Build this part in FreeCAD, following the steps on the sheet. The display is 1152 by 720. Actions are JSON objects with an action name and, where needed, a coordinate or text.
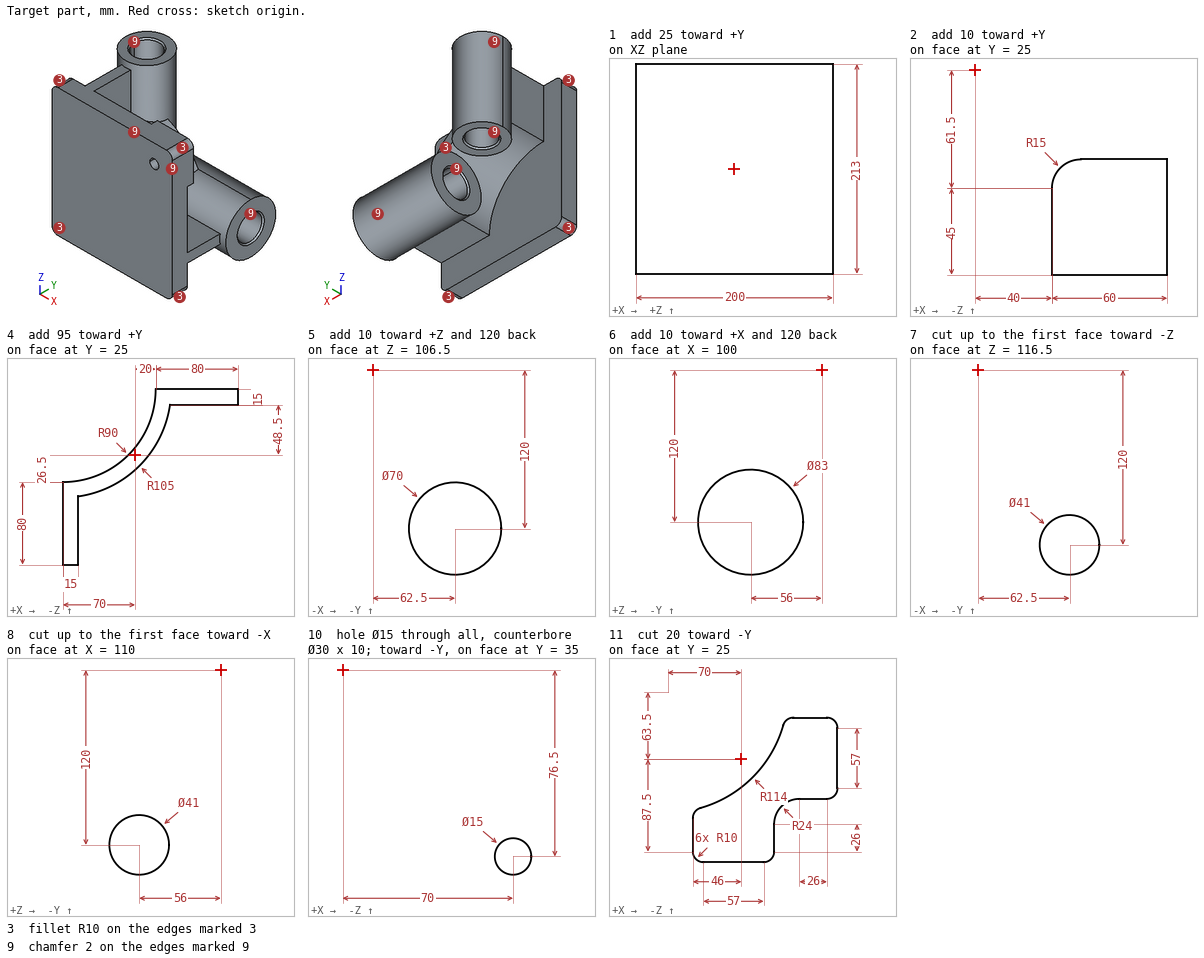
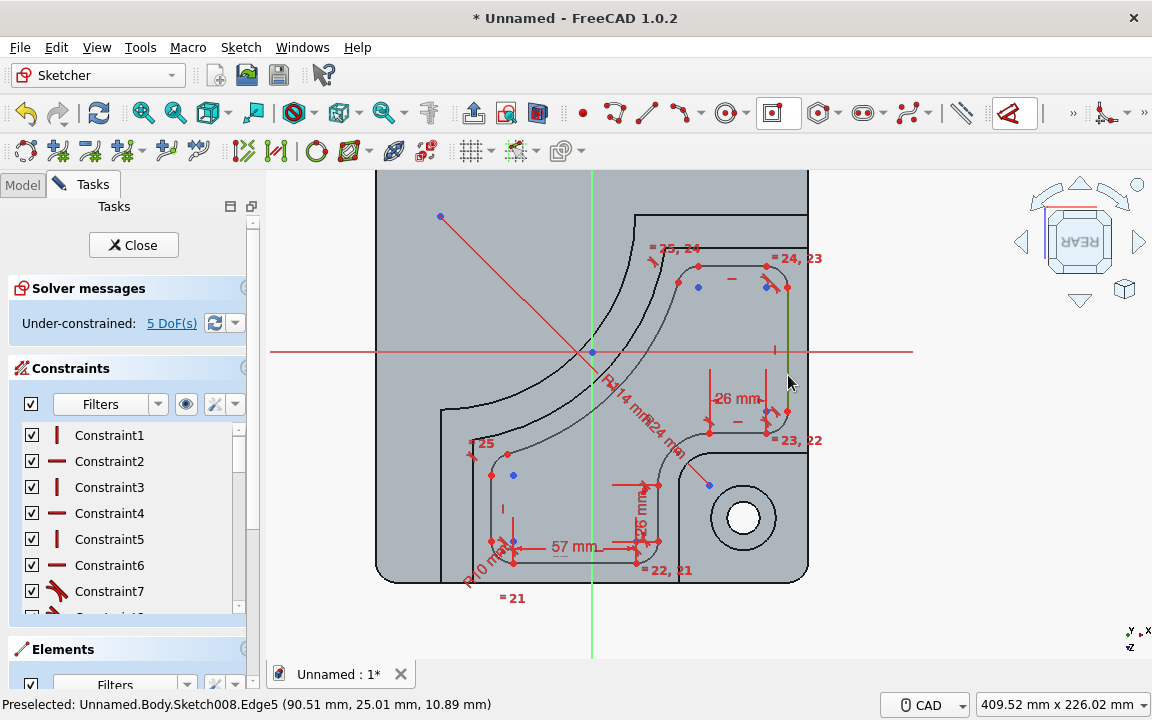
{"action": "left_click", "coordinate": [1032, 114]}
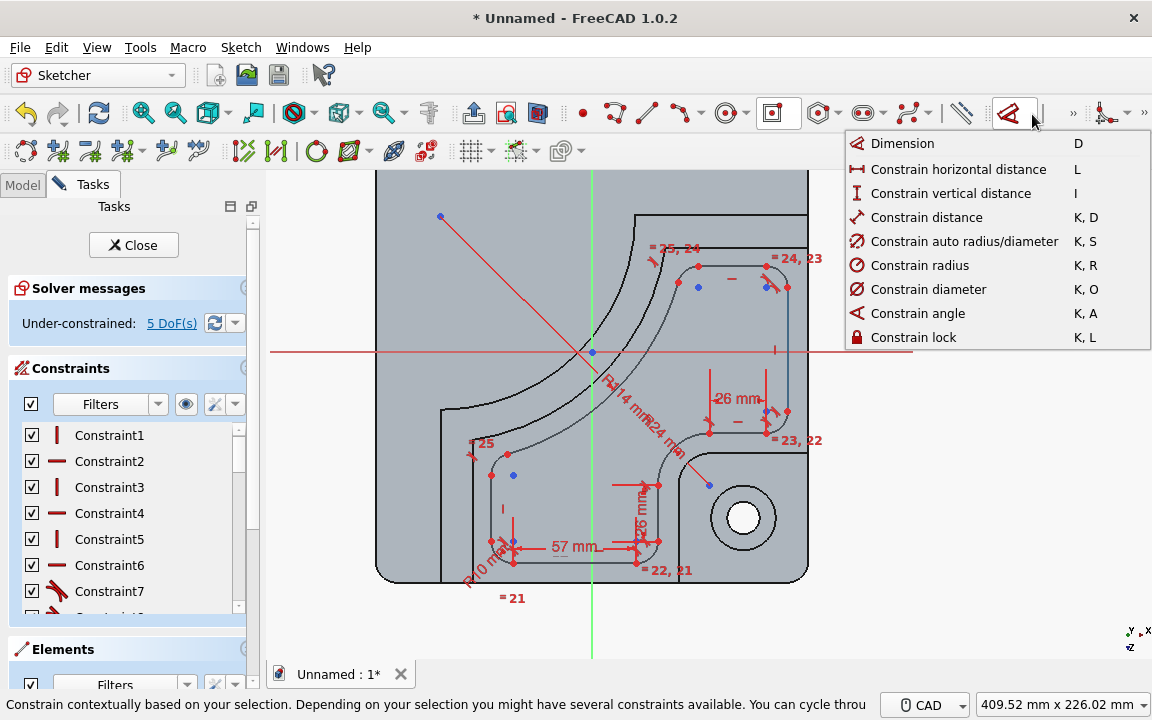
{"action": "left_click", "coordinate": [998, 193]}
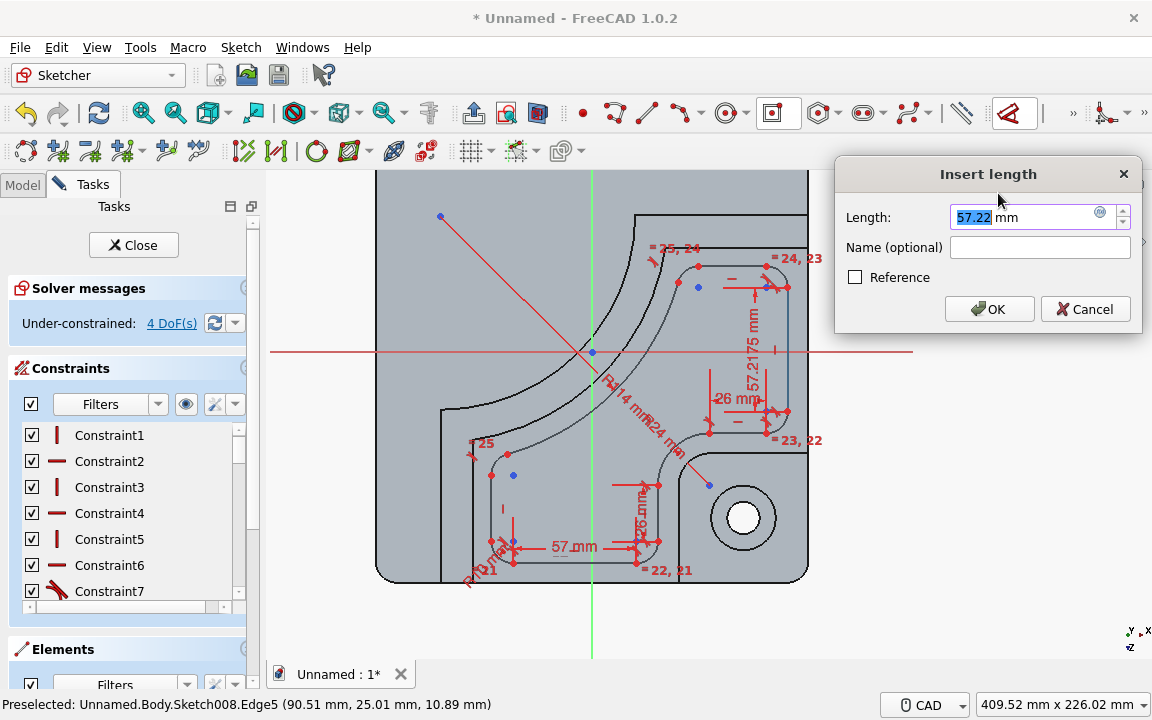
{"action": "type", "text": "57"}
{"action": "key", "text": "Return"}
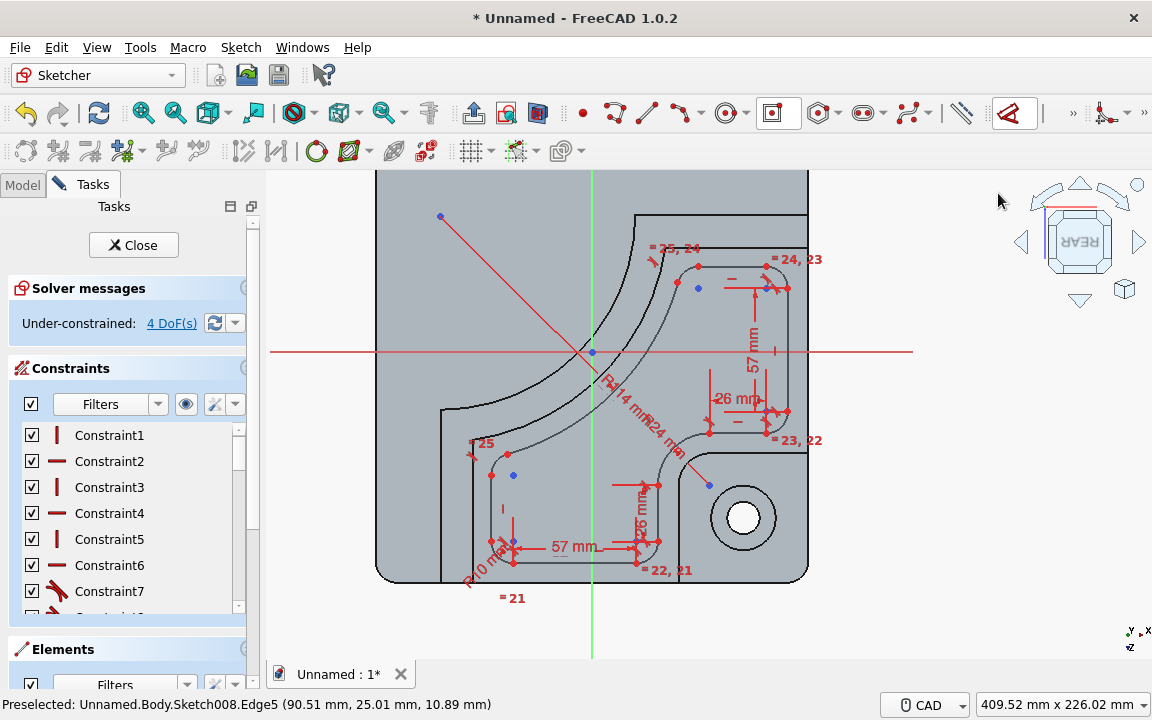
{"action": "left_click", "coordinate": [491, 475]}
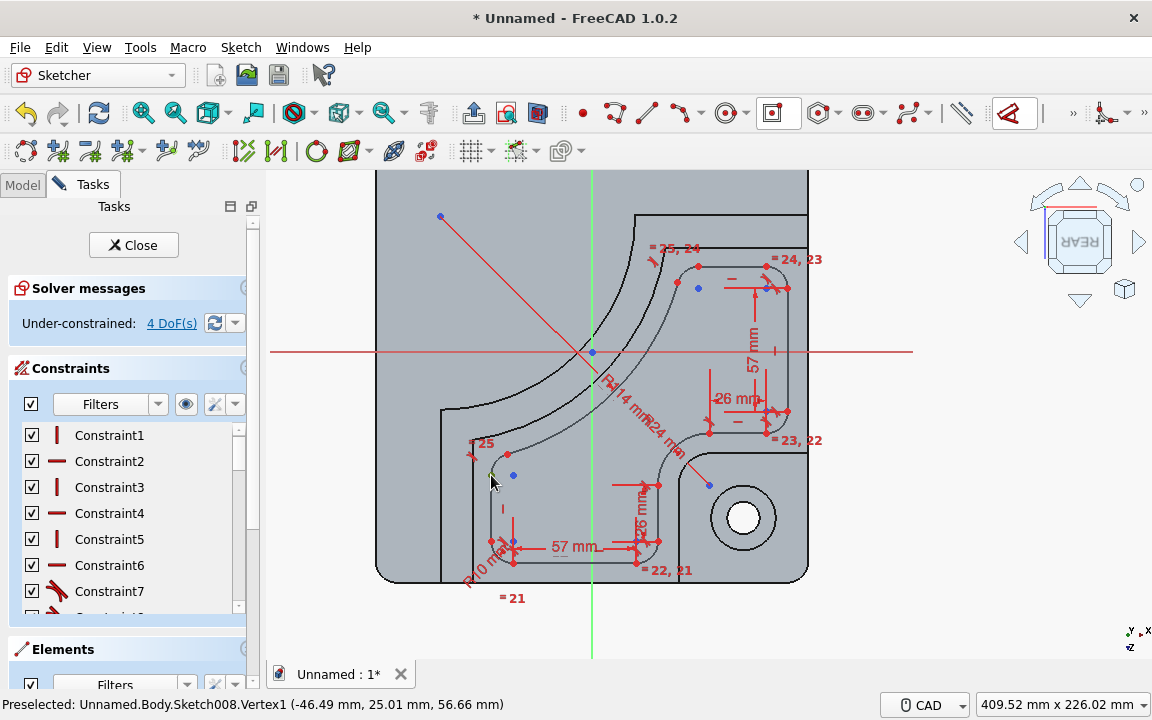
{"action": "key", "text": "l"}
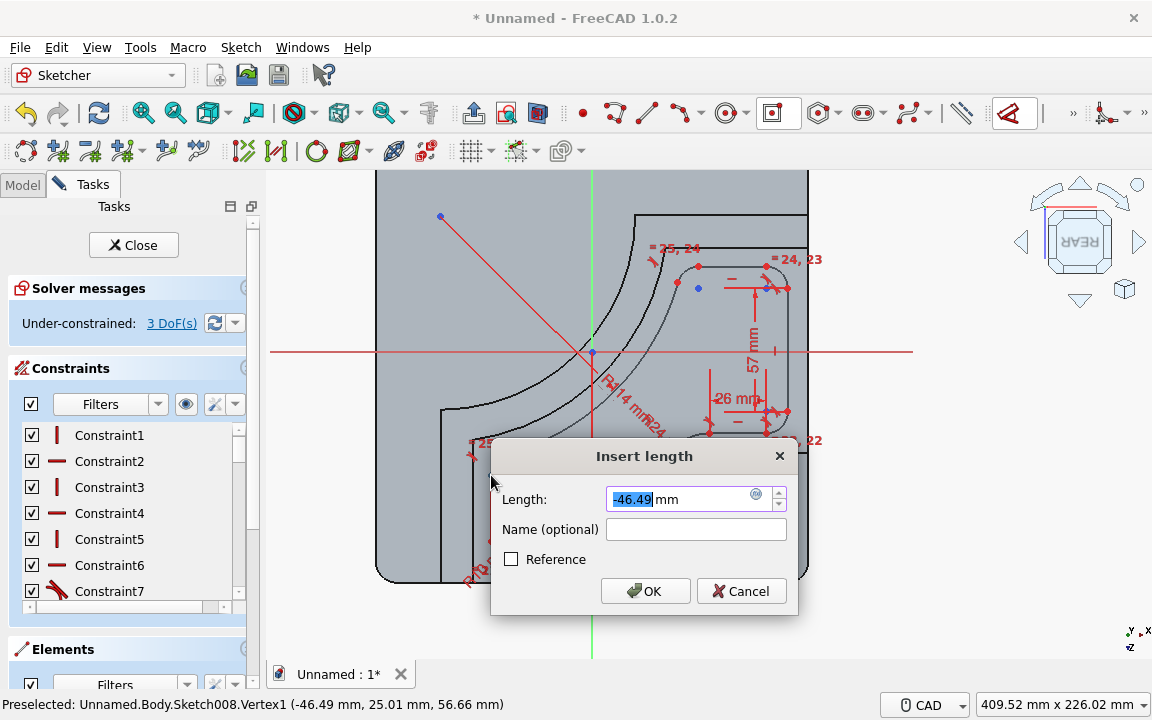
{"action": "type", "text": "-46"}
{"action": "key", "text": "Return"}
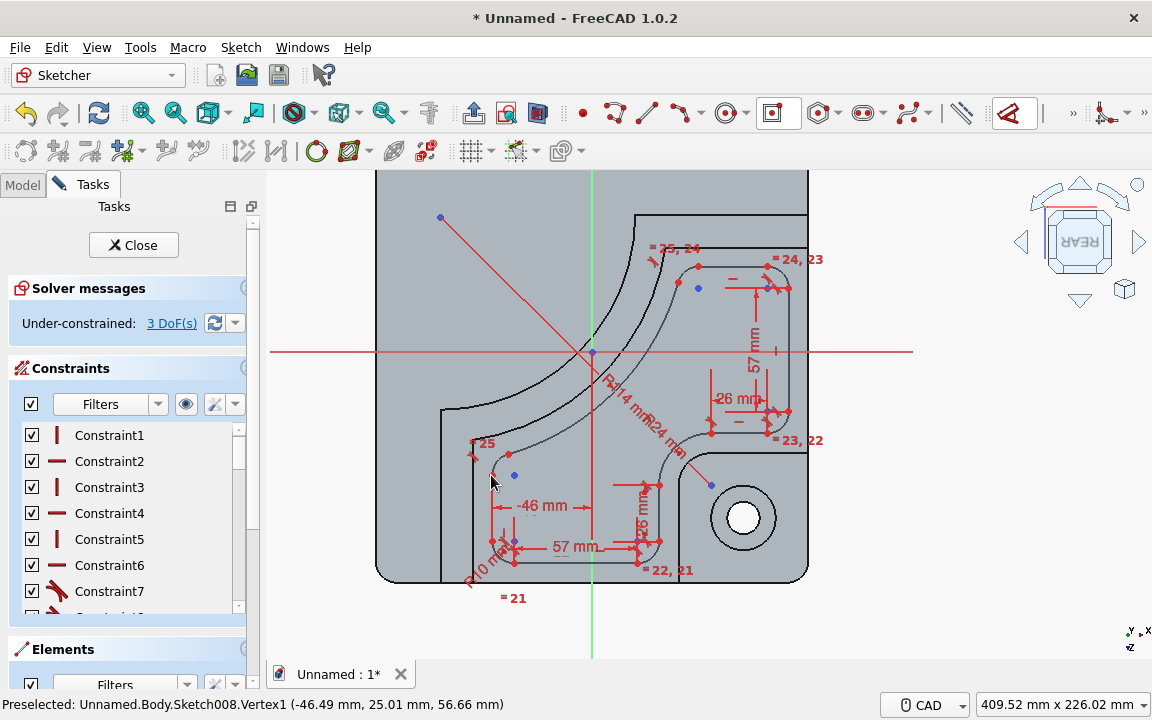
{"action": "left_click", "coordinate": [440, 217]}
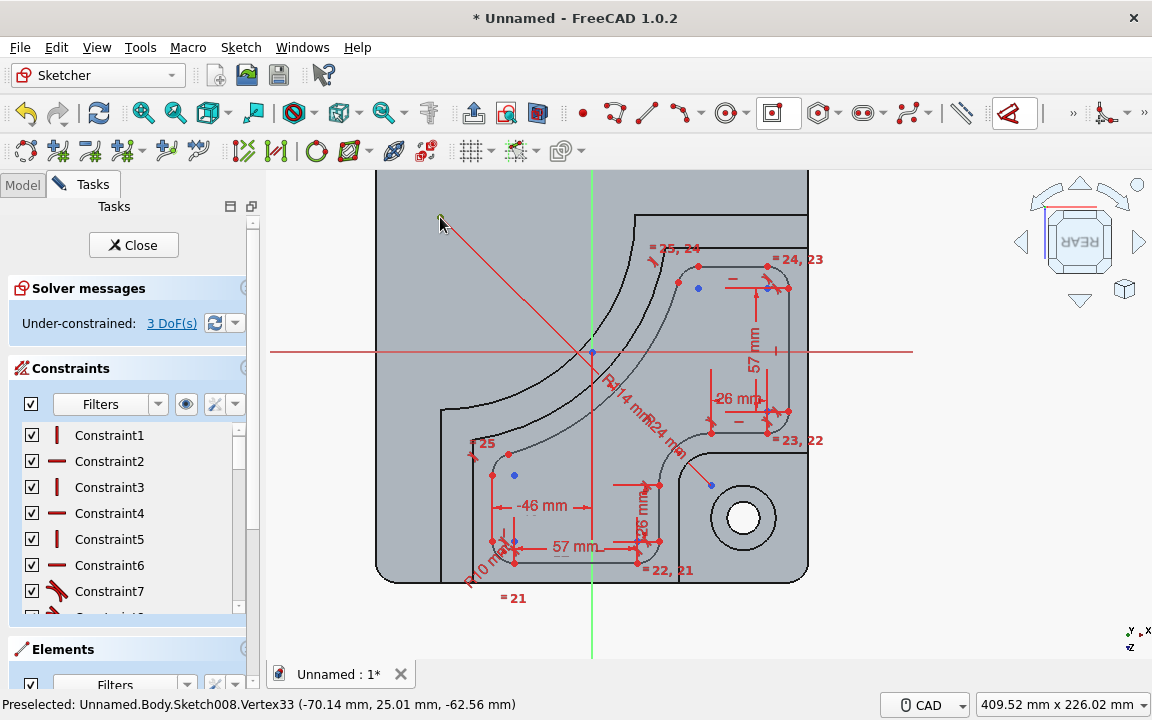
{"action": "key", "text": "l"}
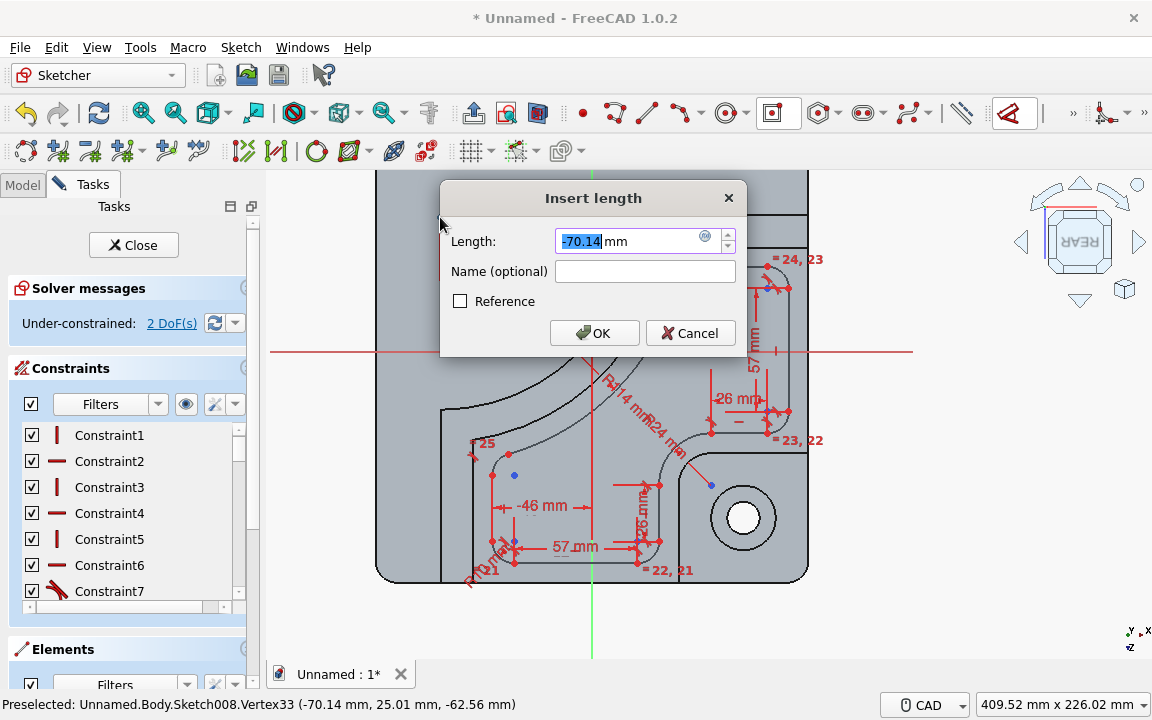
{"action": "type", "text": "-70"}
{"action": "key", "text": "Return"}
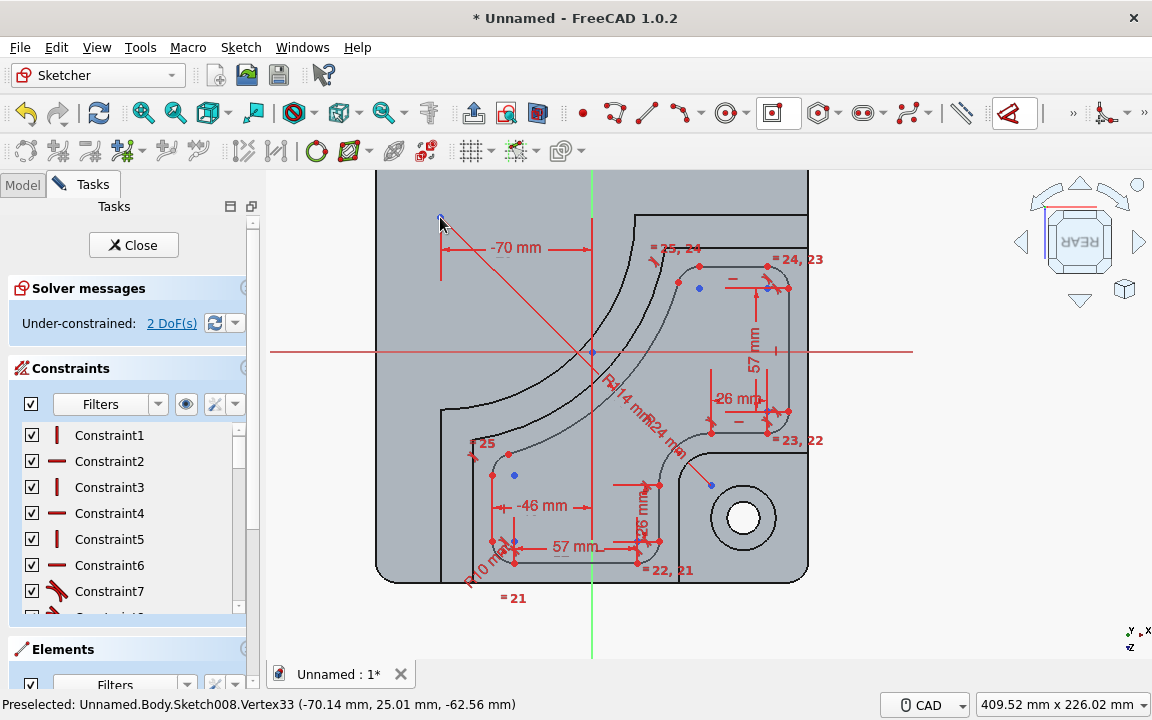
{"action": "left_click", "coordinate": [493, 542]}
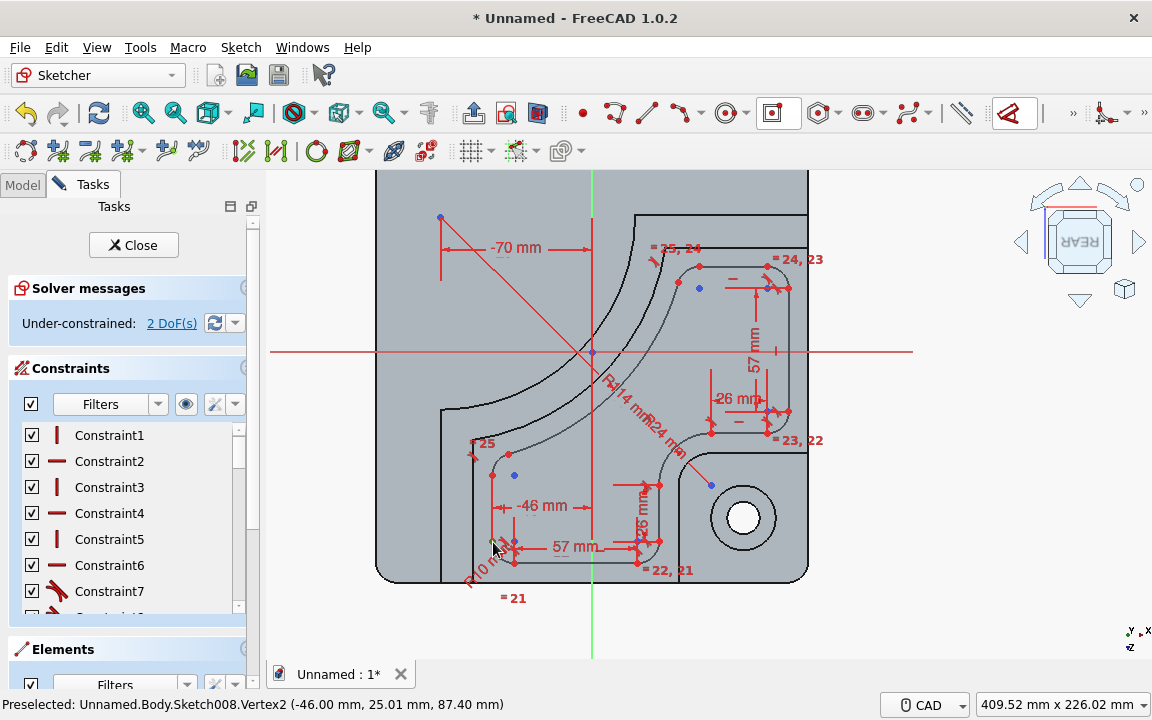
{"action": "left_click", "coordinate": [1032, 114]}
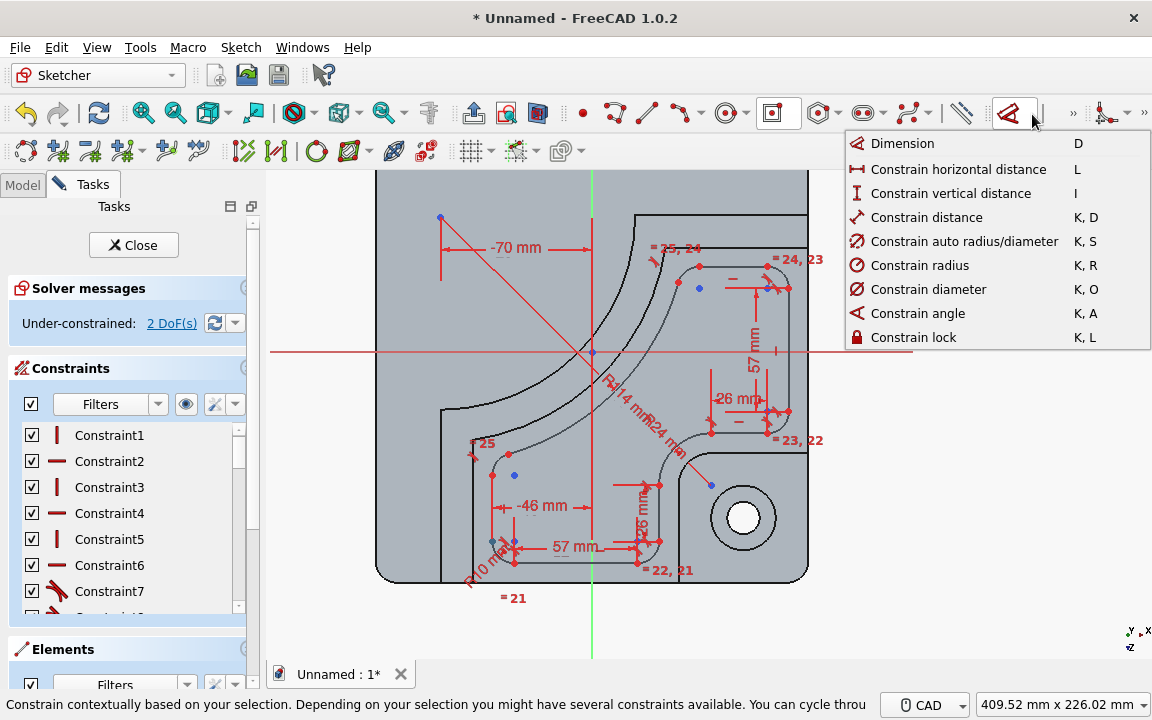
{"action": "left_click", "coordinate": [998, 193]}